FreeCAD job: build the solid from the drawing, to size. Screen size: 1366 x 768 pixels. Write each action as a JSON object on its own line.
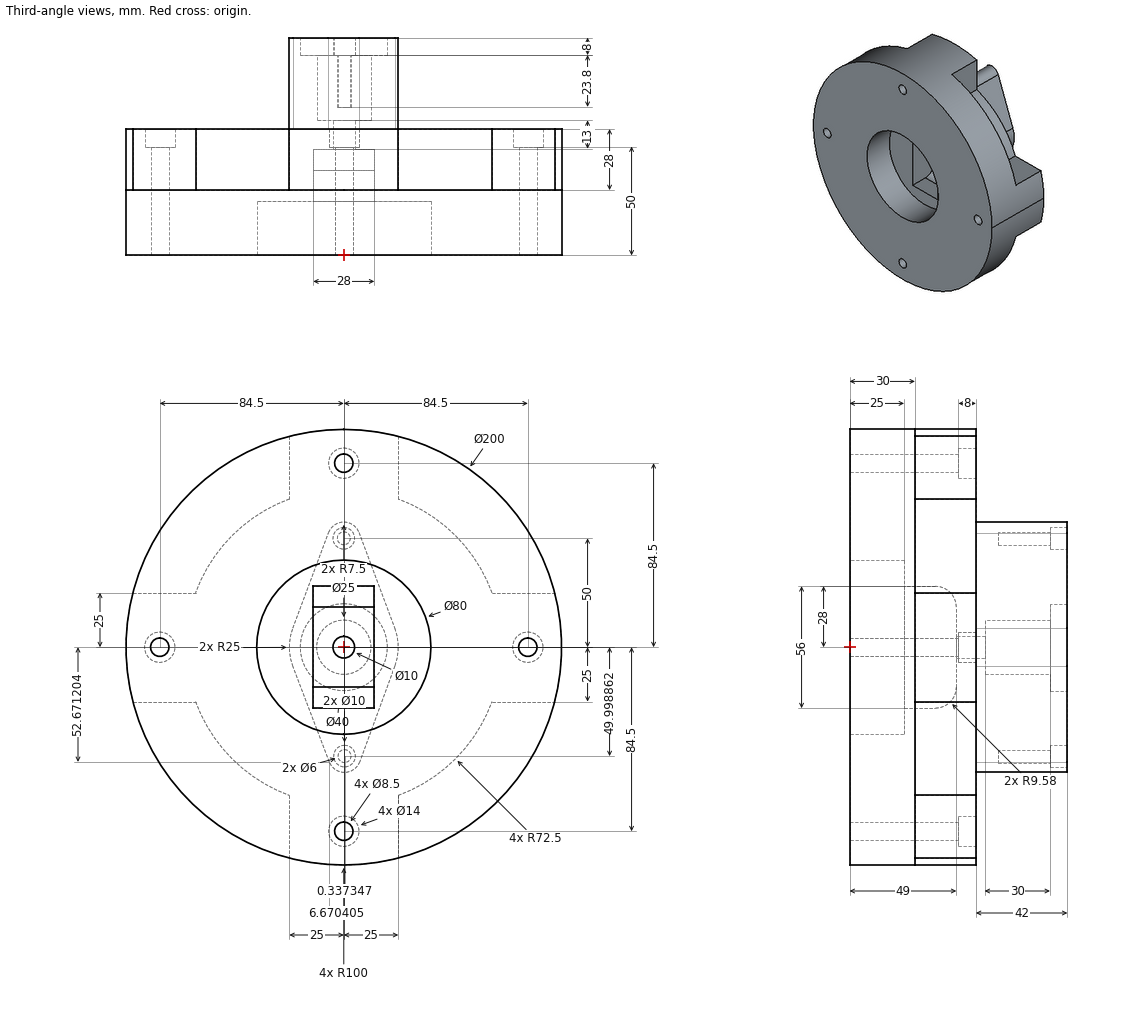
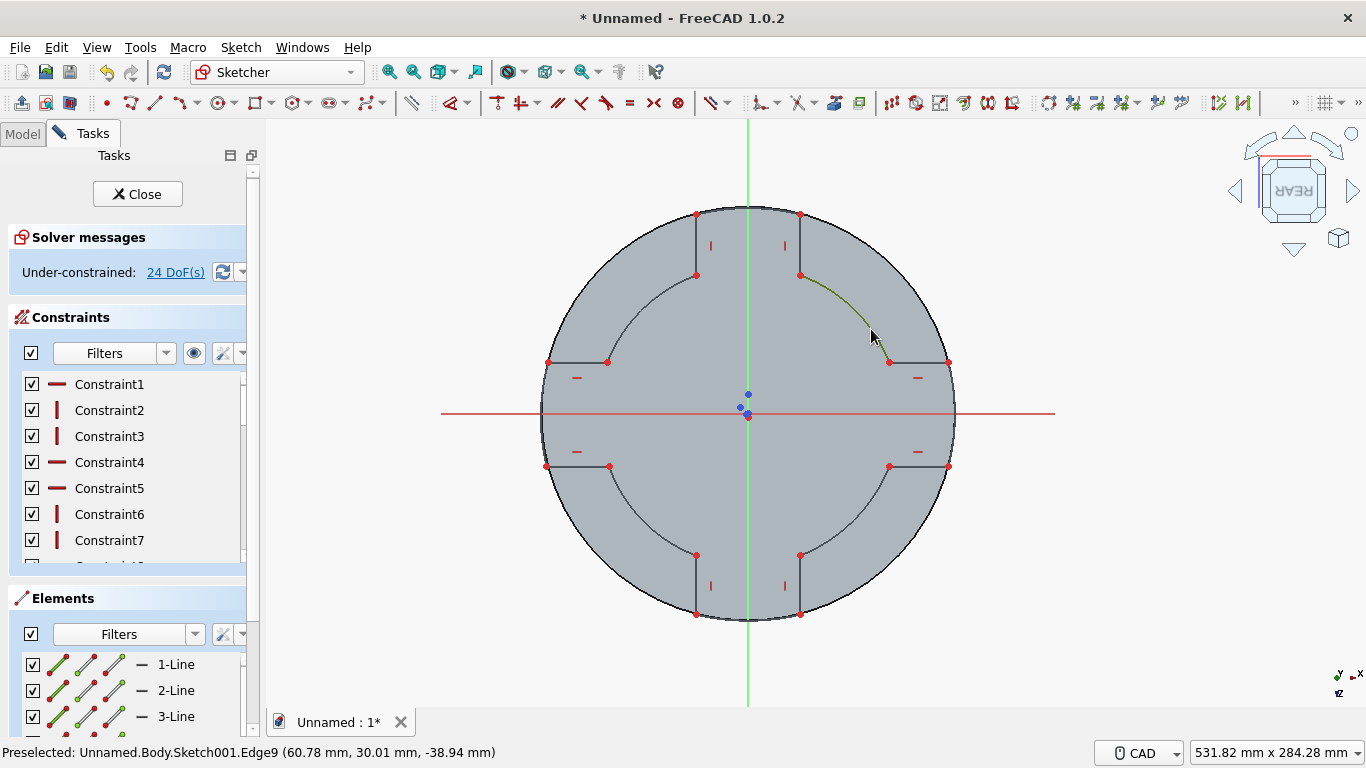
{"action": "left_click", "coordinate": [727, 620]}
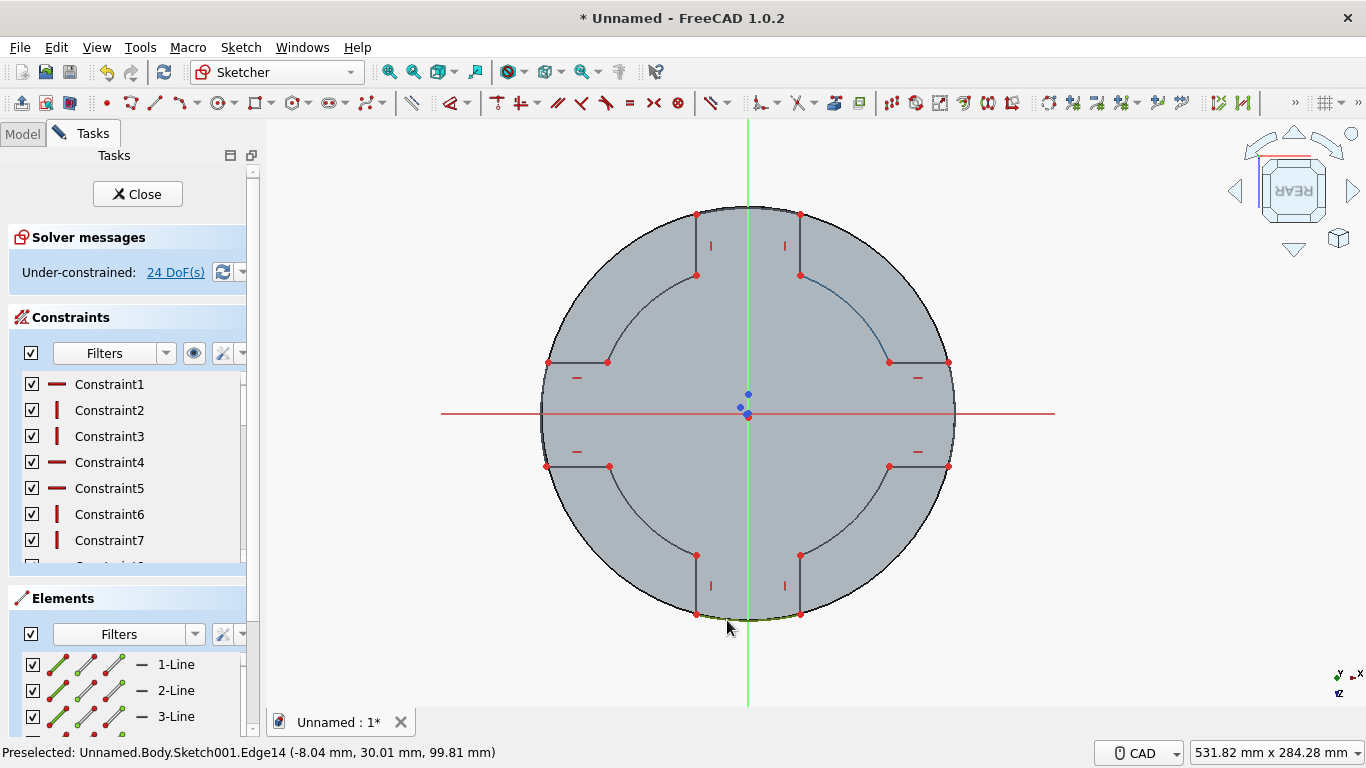
{"action": "left_click", "coordinate": [498, 104]}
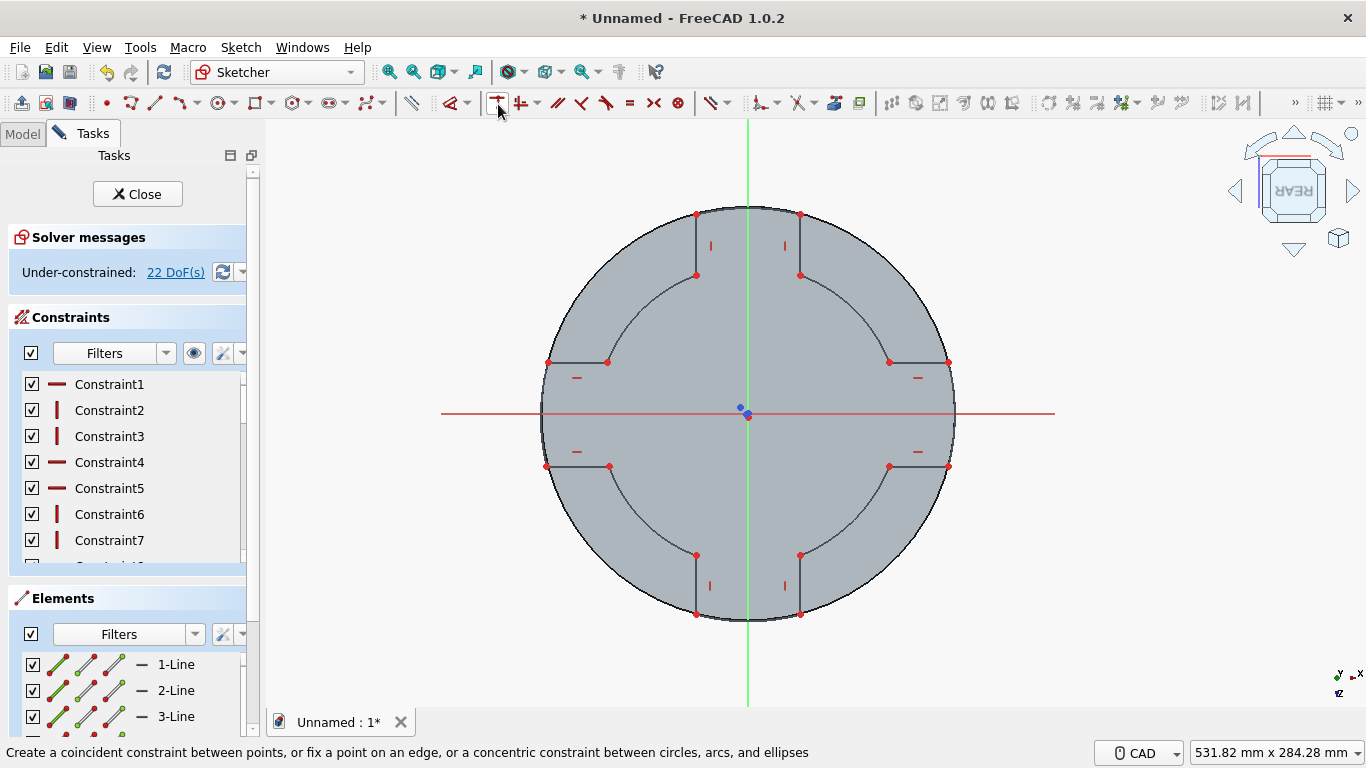
{"action": "left_click", "coordinate": [871, 329]}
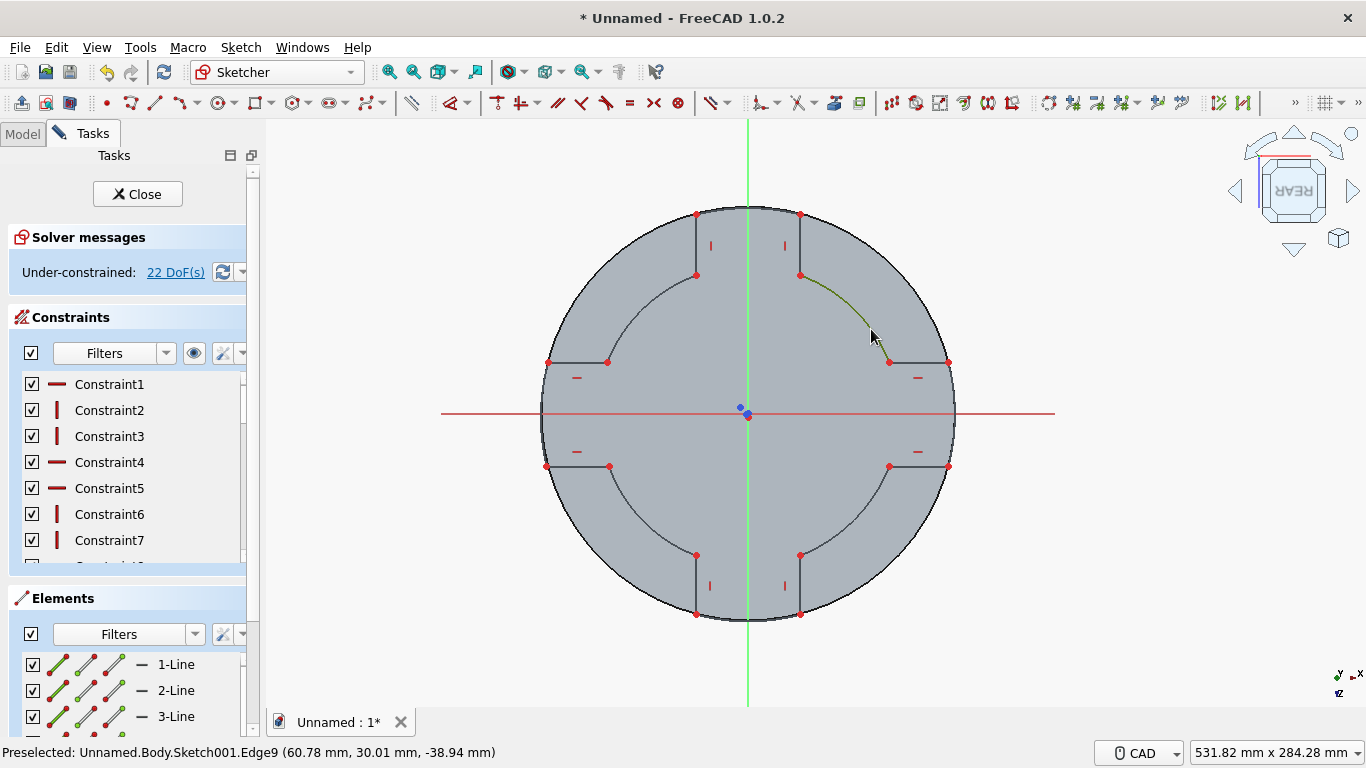
{"action": "left_click", "coordinate": [834, 537]}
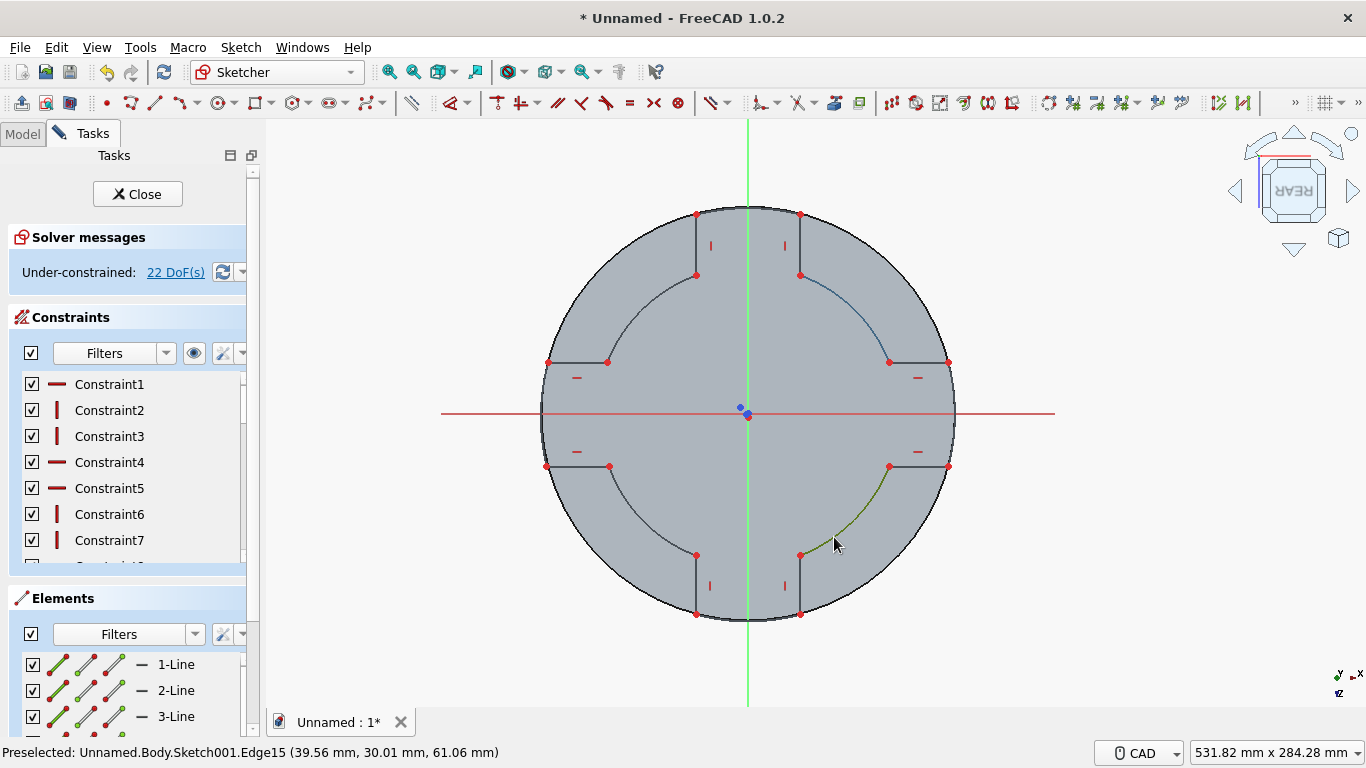
{"action": "key", "text": "c"}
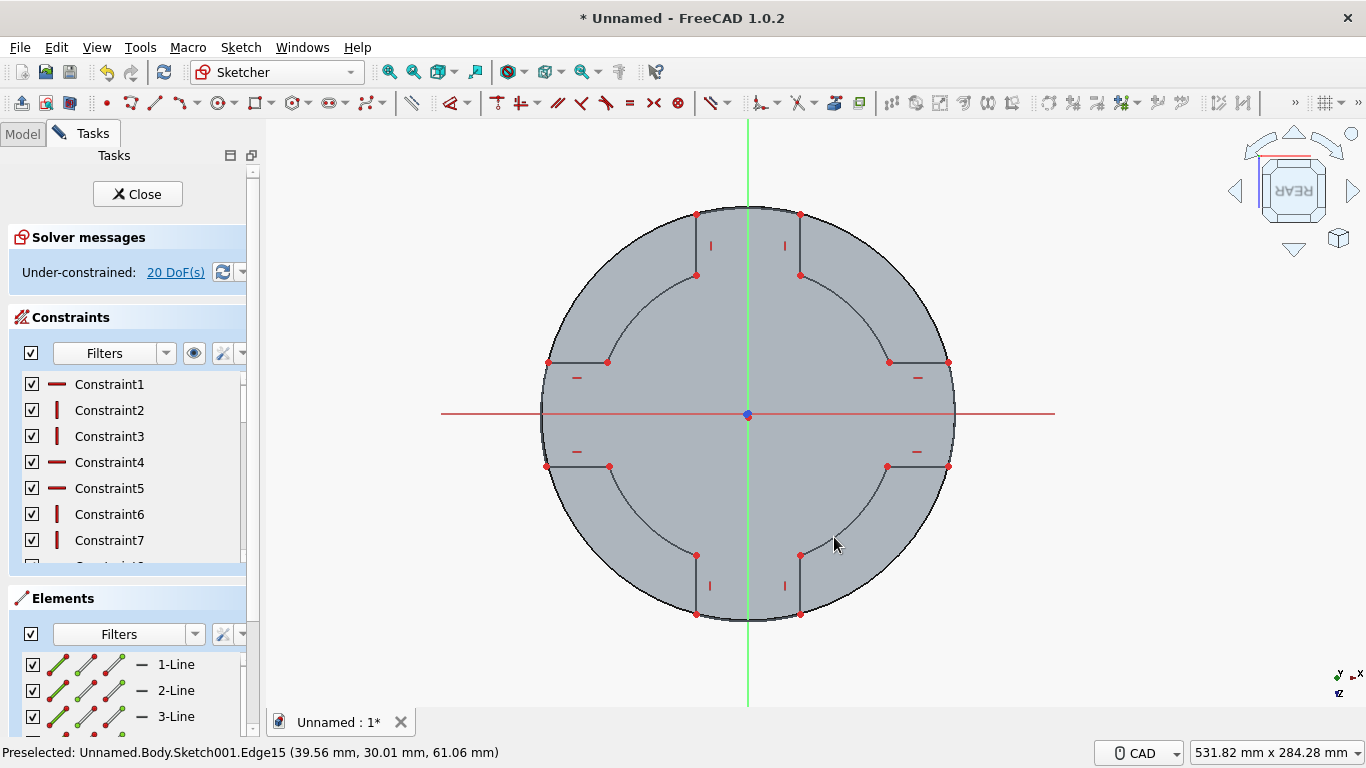
{"action": "left_click", "coordinate": [871, 329]}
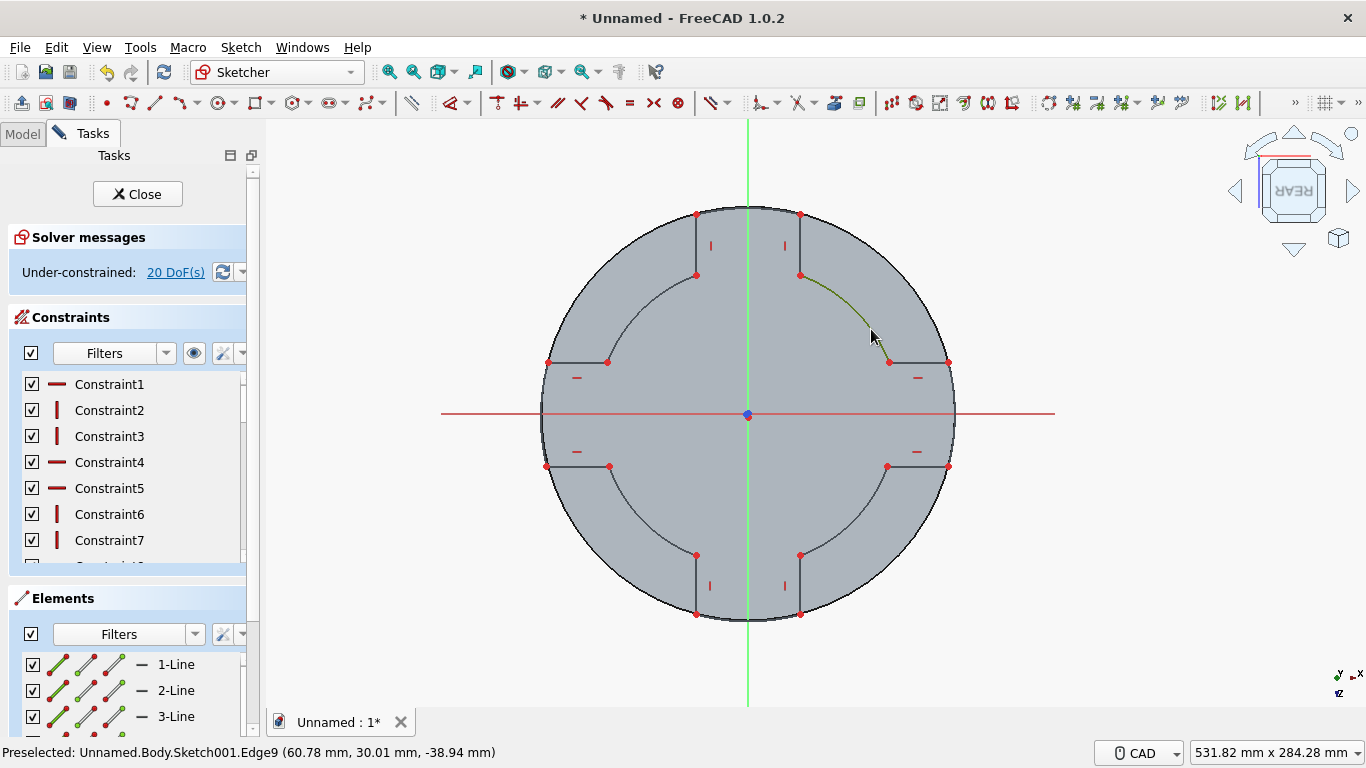
{"action": "left_click", "coordinate": [954, 436]}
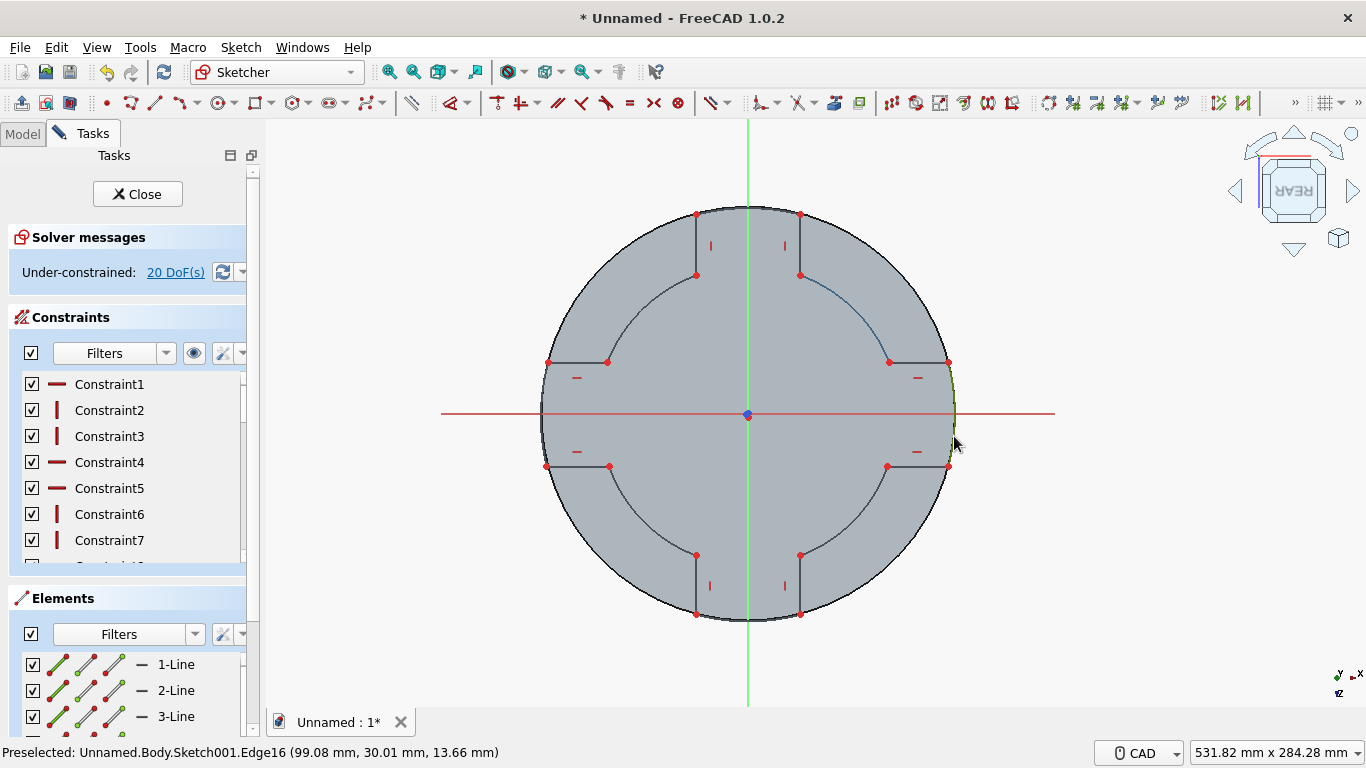
{"action": "left_click", "coordinate": [498, 104]}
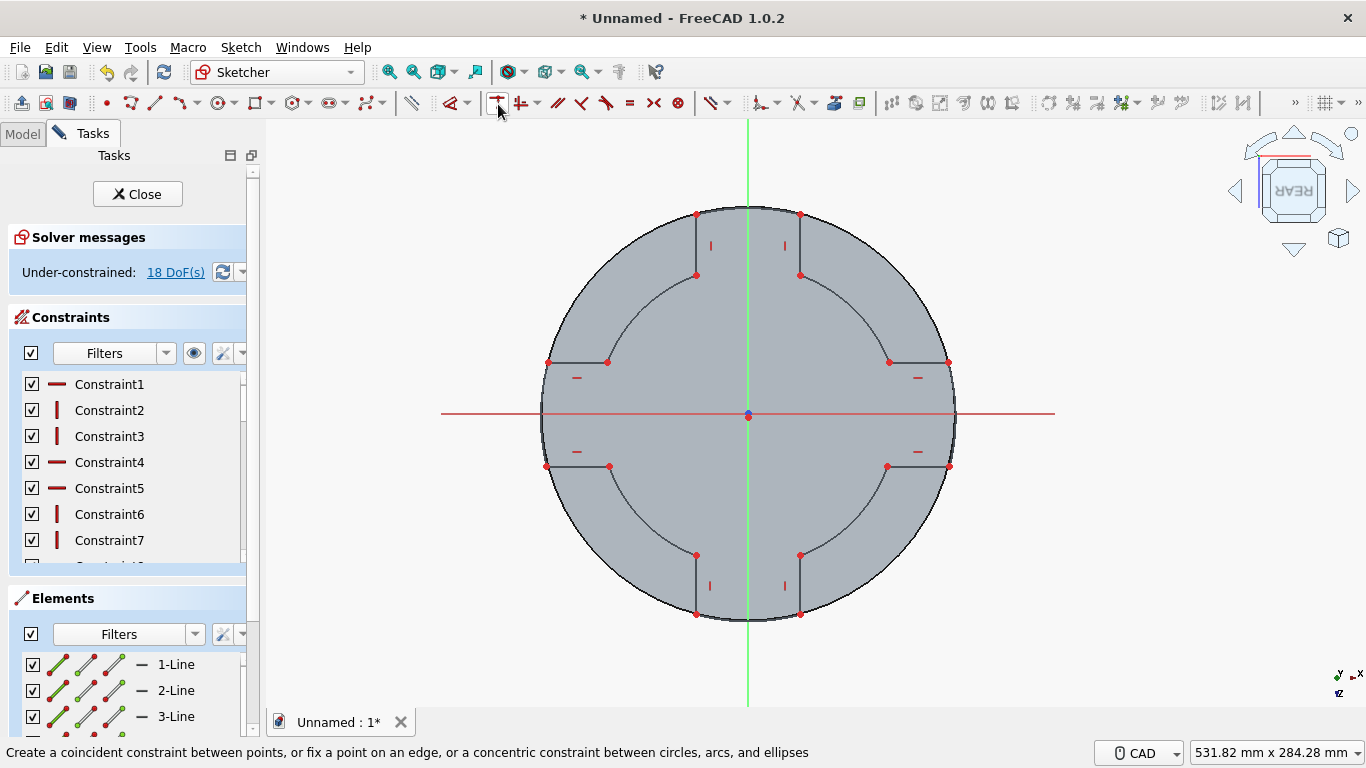
{"action": "left_click_drag", "start_coordinate": [738, 404], "coordinate": [758, 428]}